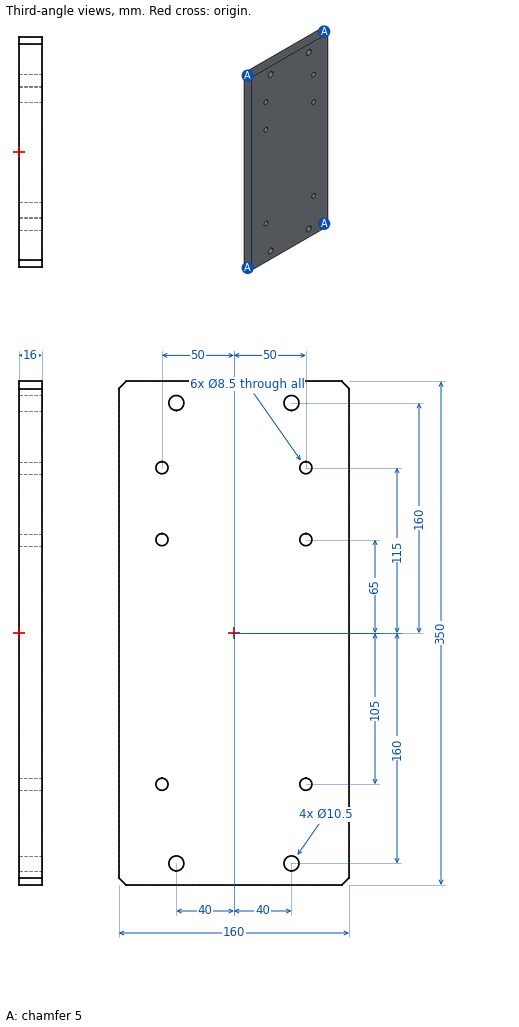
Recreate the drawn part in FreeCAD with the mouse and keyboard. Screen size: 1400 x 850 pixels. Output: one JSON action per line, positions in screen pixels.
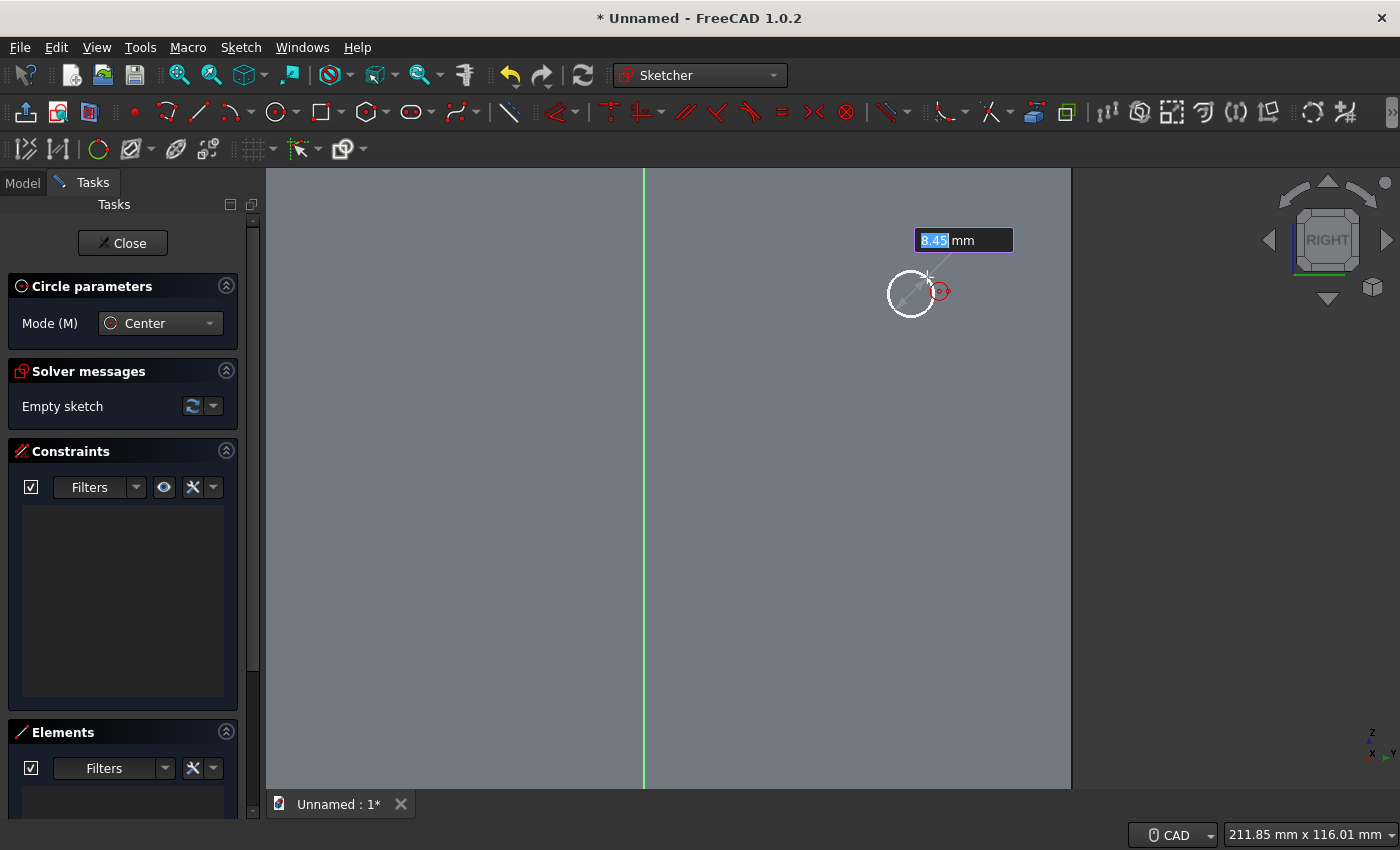
{"action": "type", "text": "8.5"}
{"action": "key", "text": "Return"}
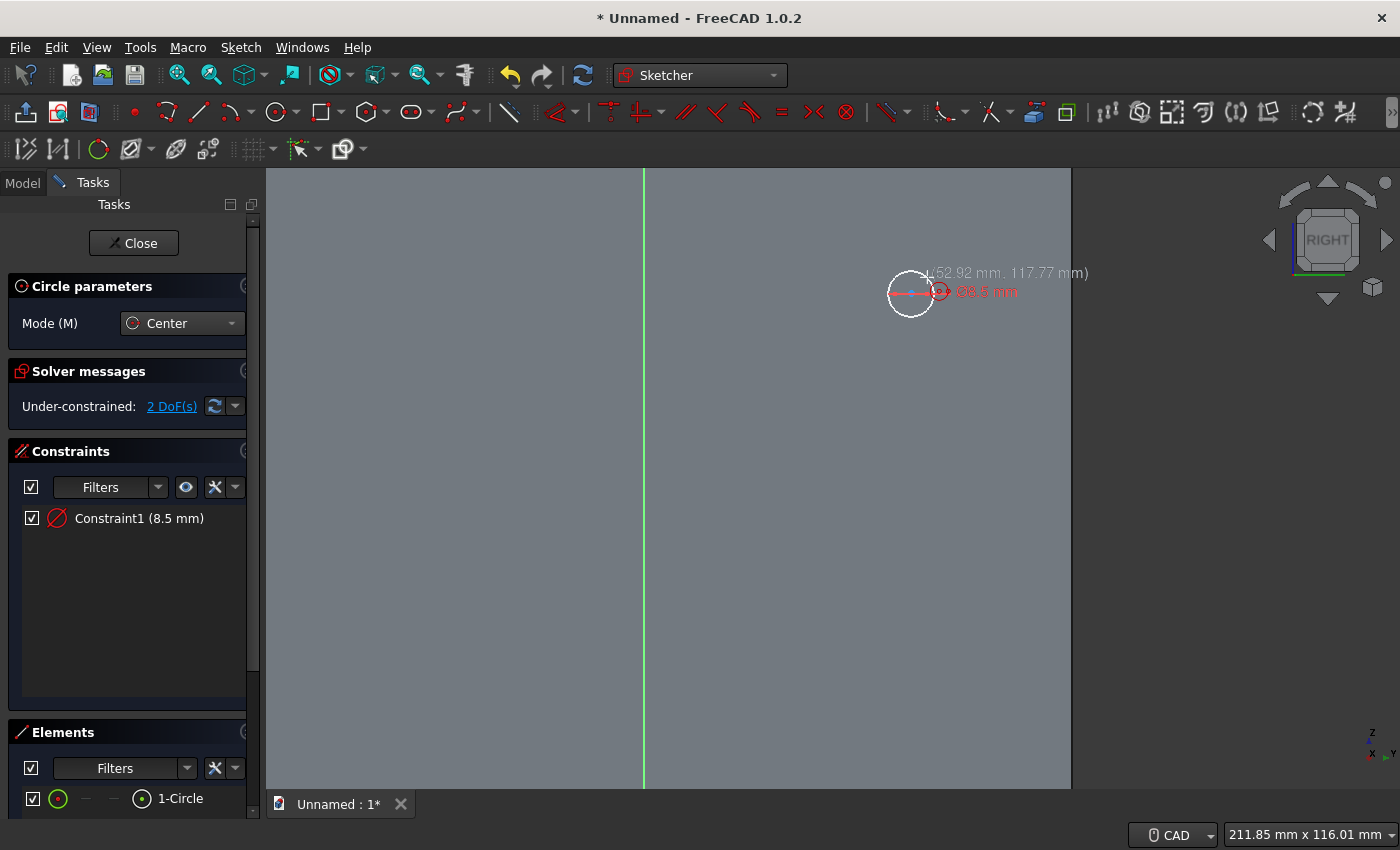
{"action": "left_click", "coordinate": [376, 293]}
{"action": "mouse_move", "coordinate": [392, 277]}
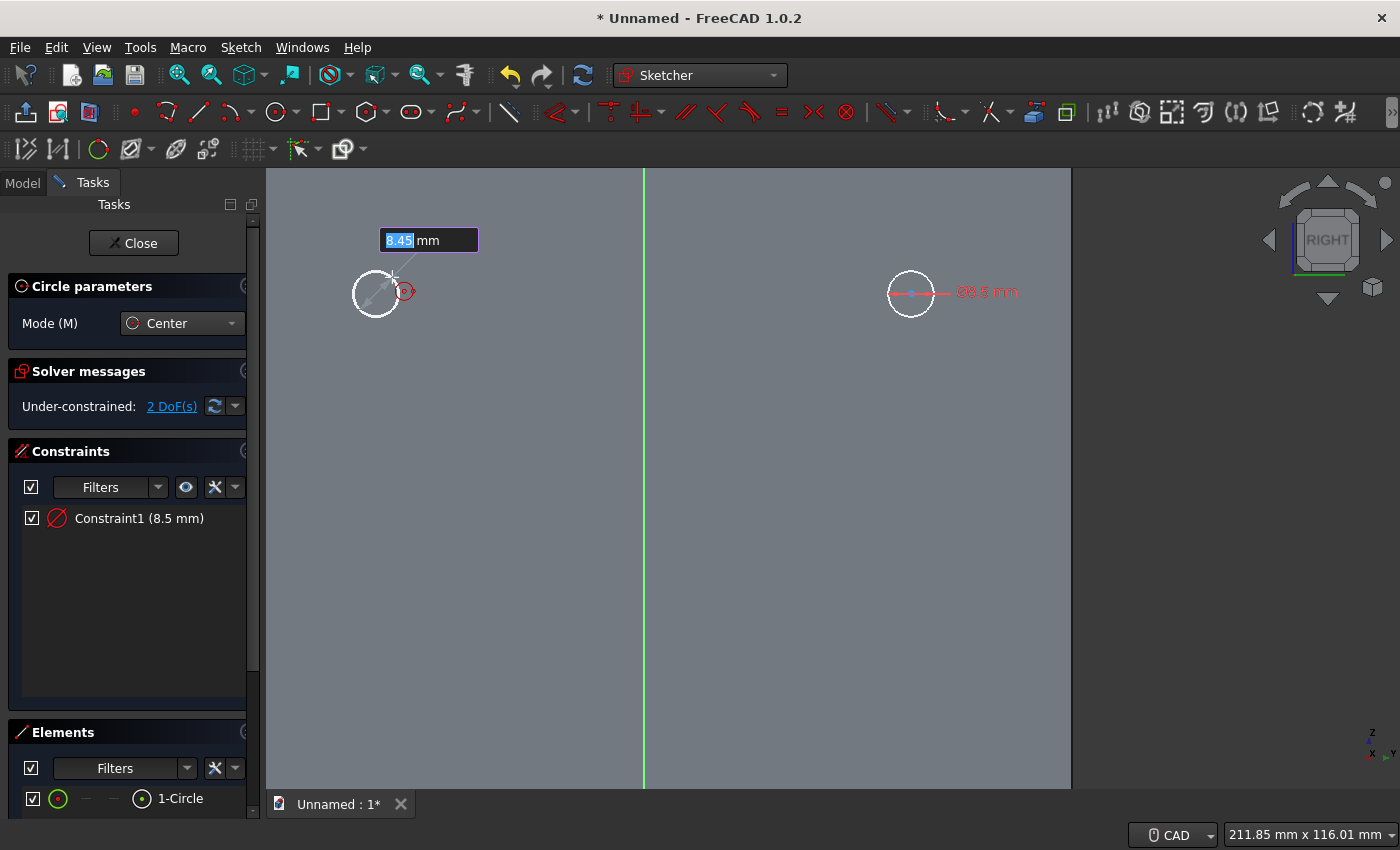
{"action": "type", "text": "8.5"}
{"action": "key", "text": "Return"}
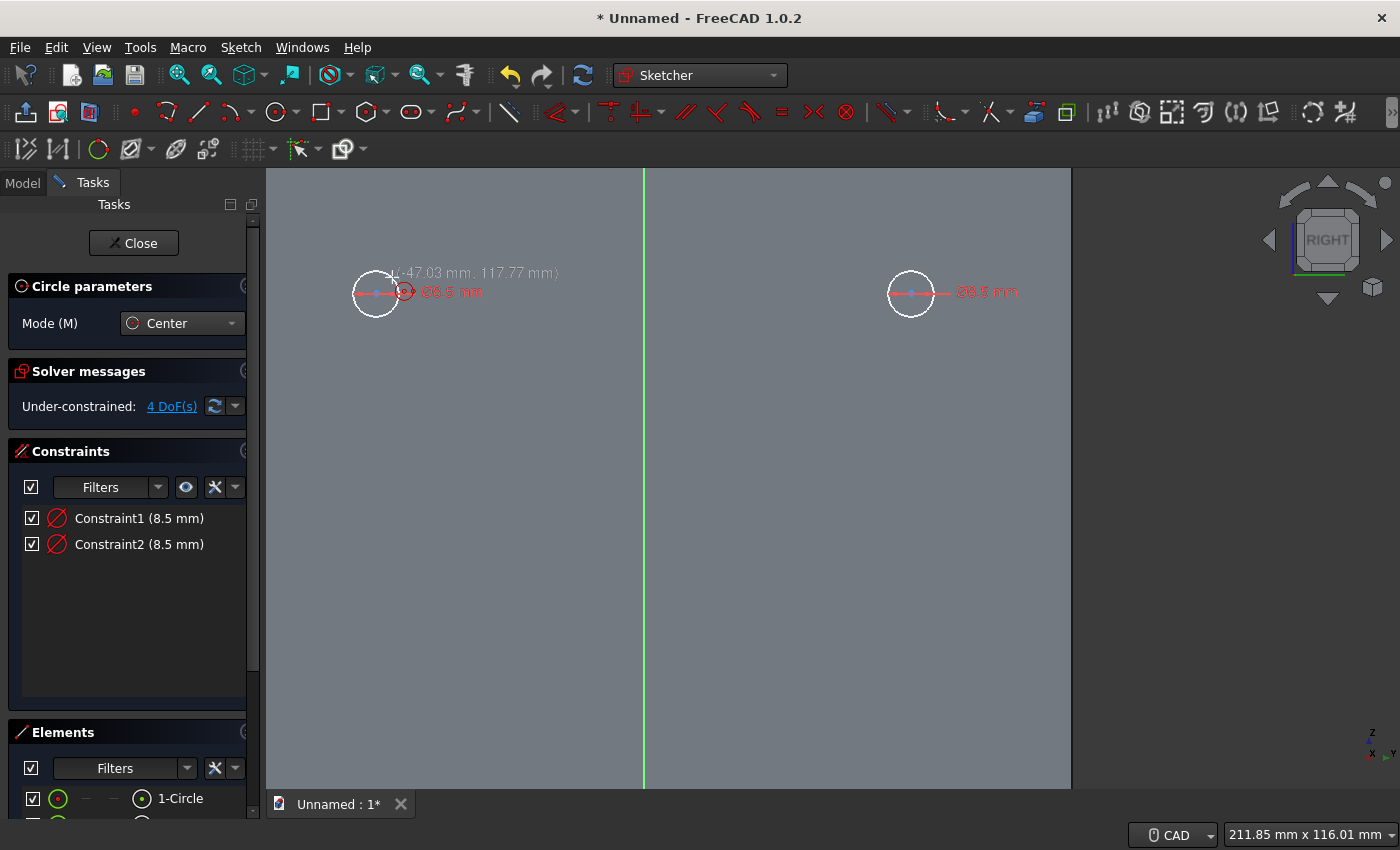
{"action": "scroll", "coordinate": [817, 305], "scroll_direction": "down", "scroll_amount": 6}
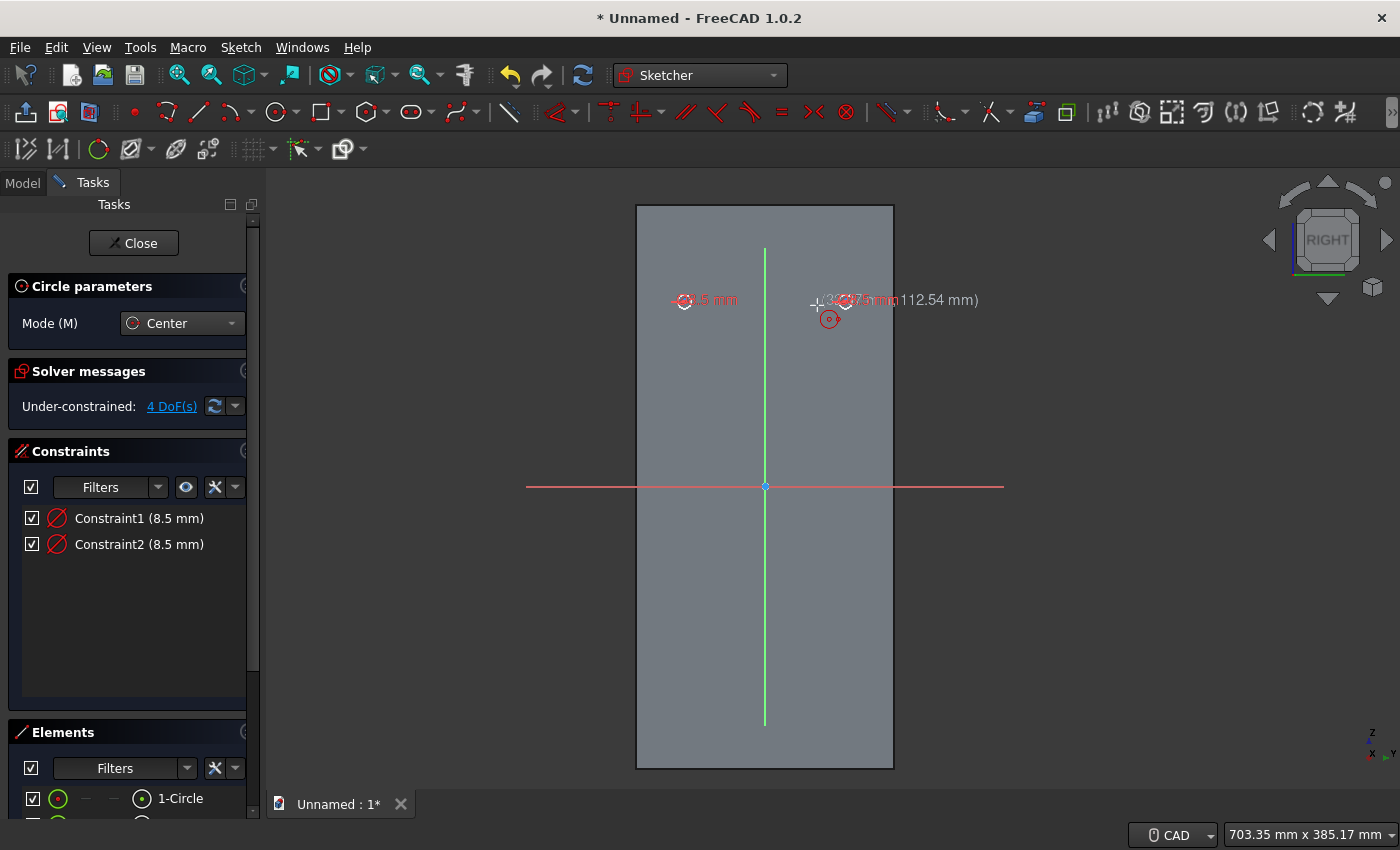
{"action": "scroll", "coordinate": [846, 656], "scroll_direction": "up", "scroll_amount": 6}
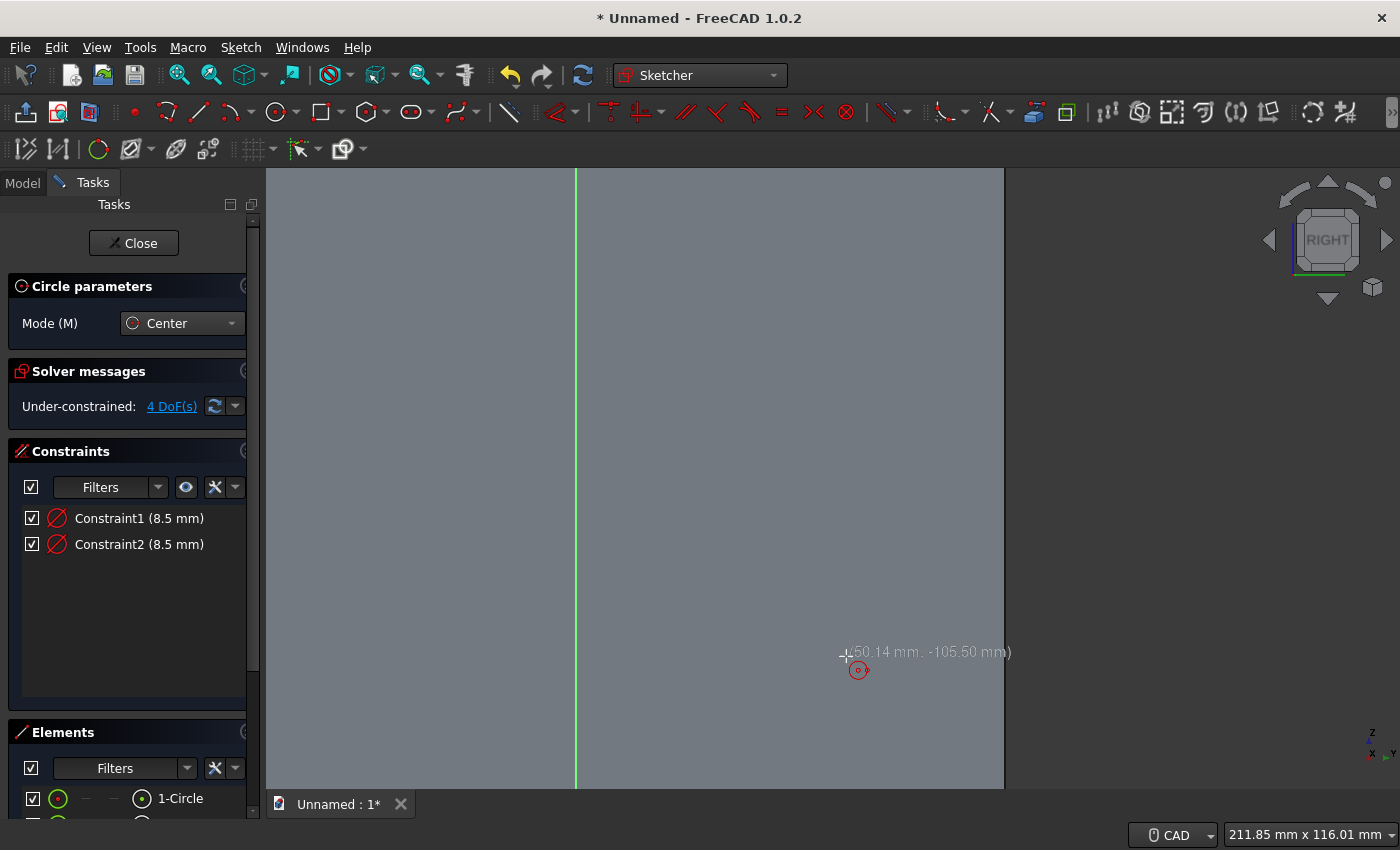
{"action": "left_click", "coordinate": [844, 655]}
{"action": "mouse_move", "coordinate": [860, 639]}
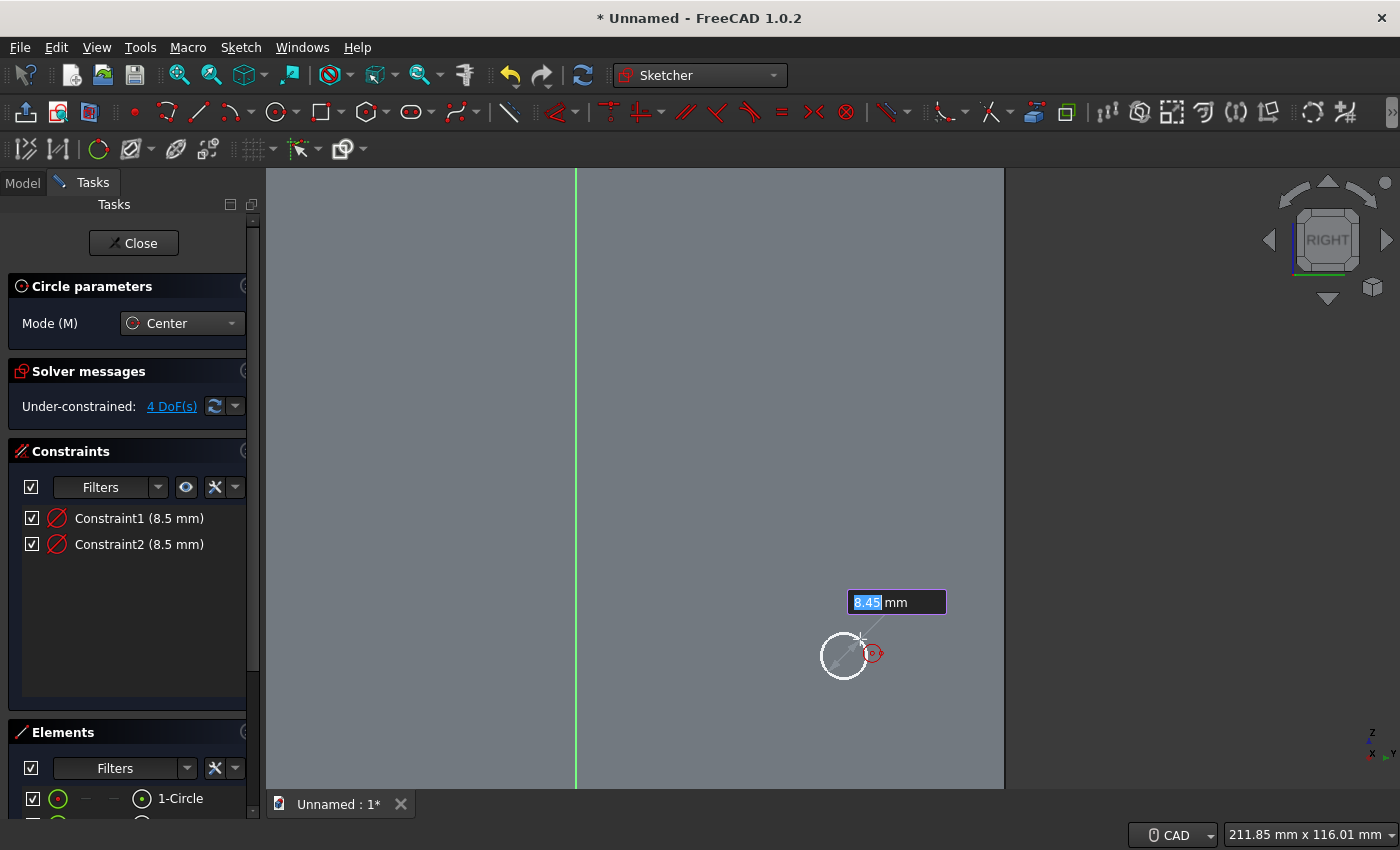
{"action": "type", "text": "8.5"}
{"action": "key", "text": "Return"}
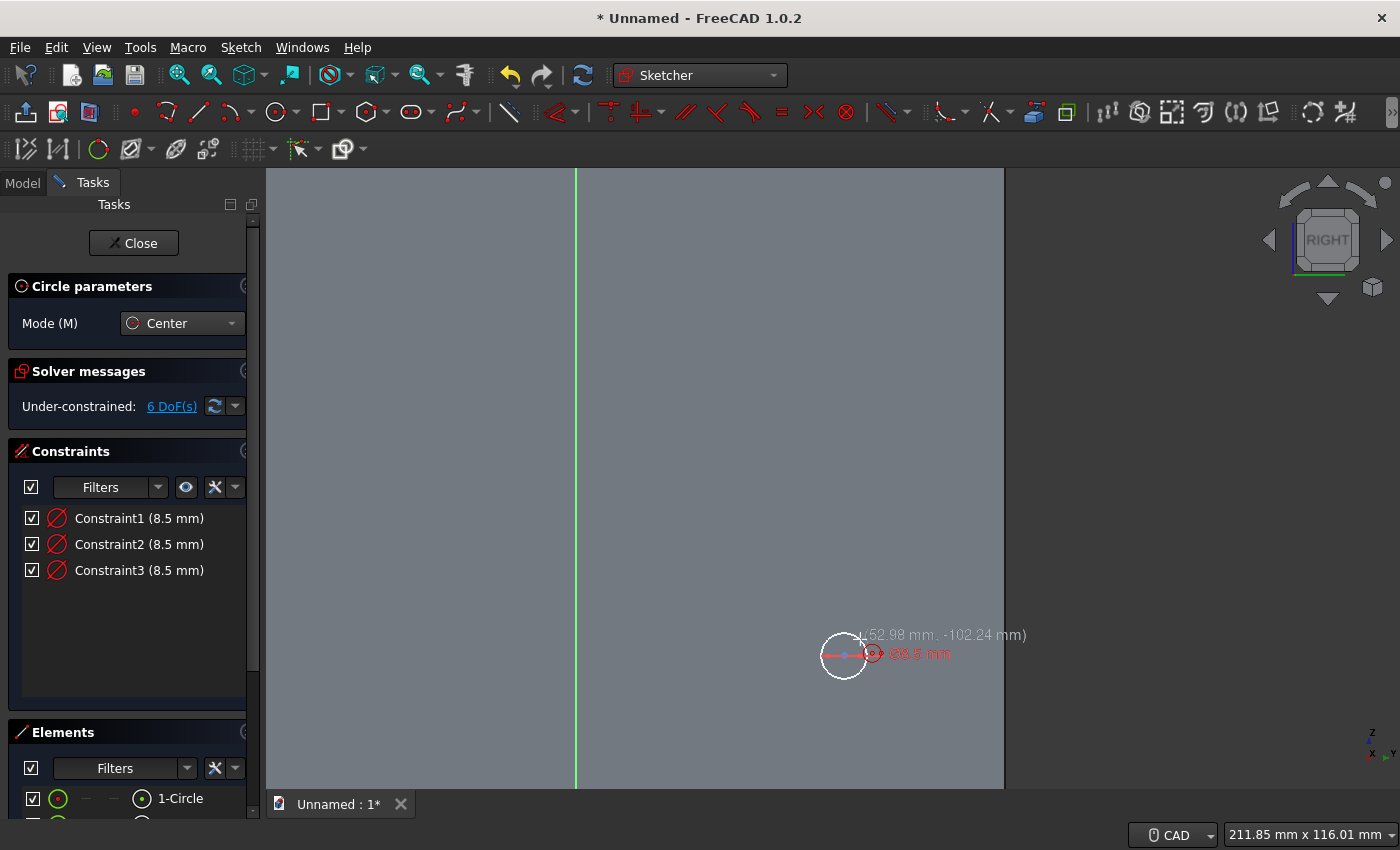
{"action": "left_click", "coordinate": [309, 655]}
{"action": "mouse_move", "coordinate": [325, 639]}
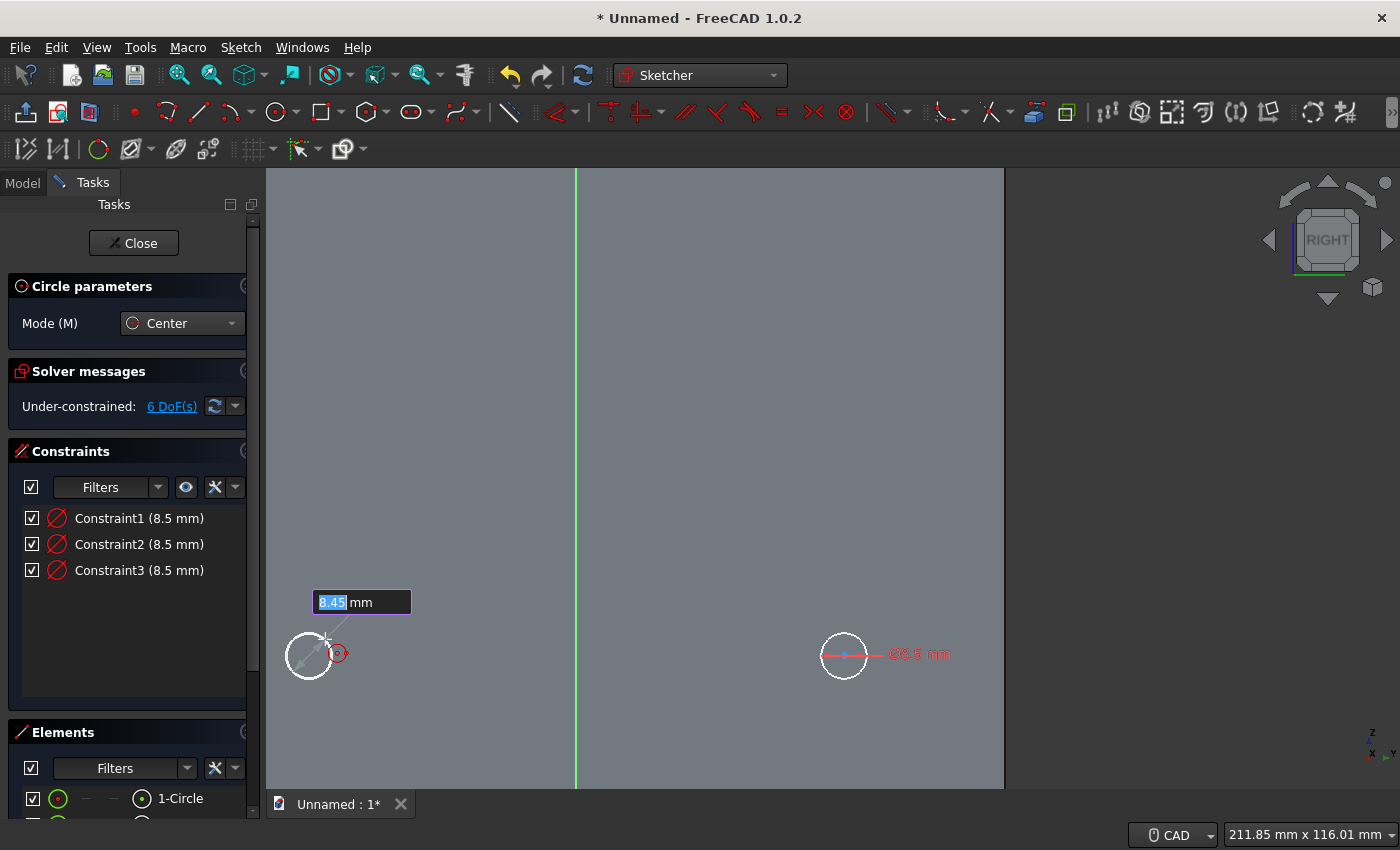
{"action": "type", "text": "8.5"}
{"action": "key", "text": "Return"}